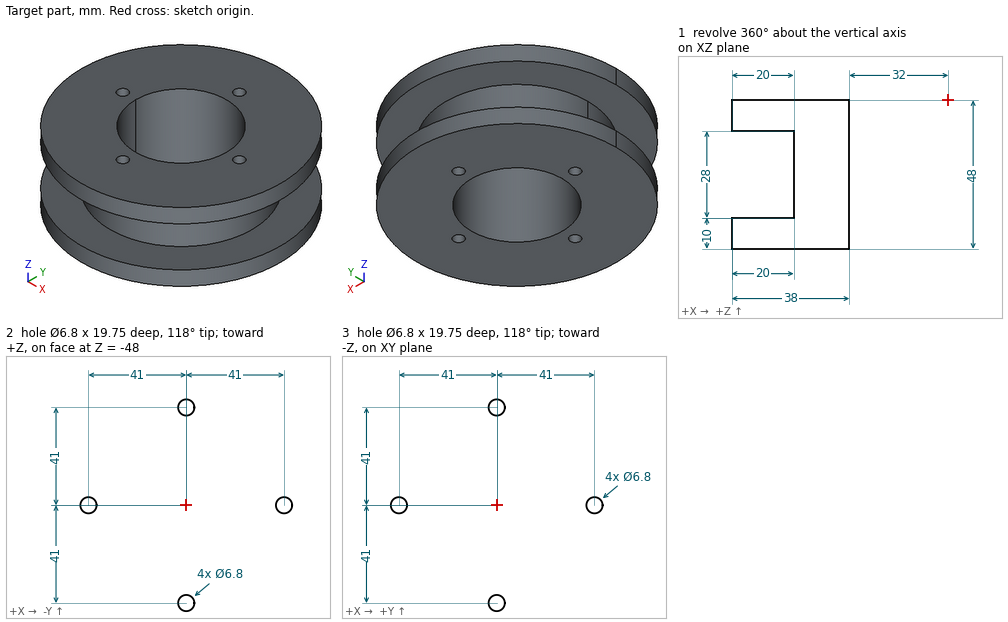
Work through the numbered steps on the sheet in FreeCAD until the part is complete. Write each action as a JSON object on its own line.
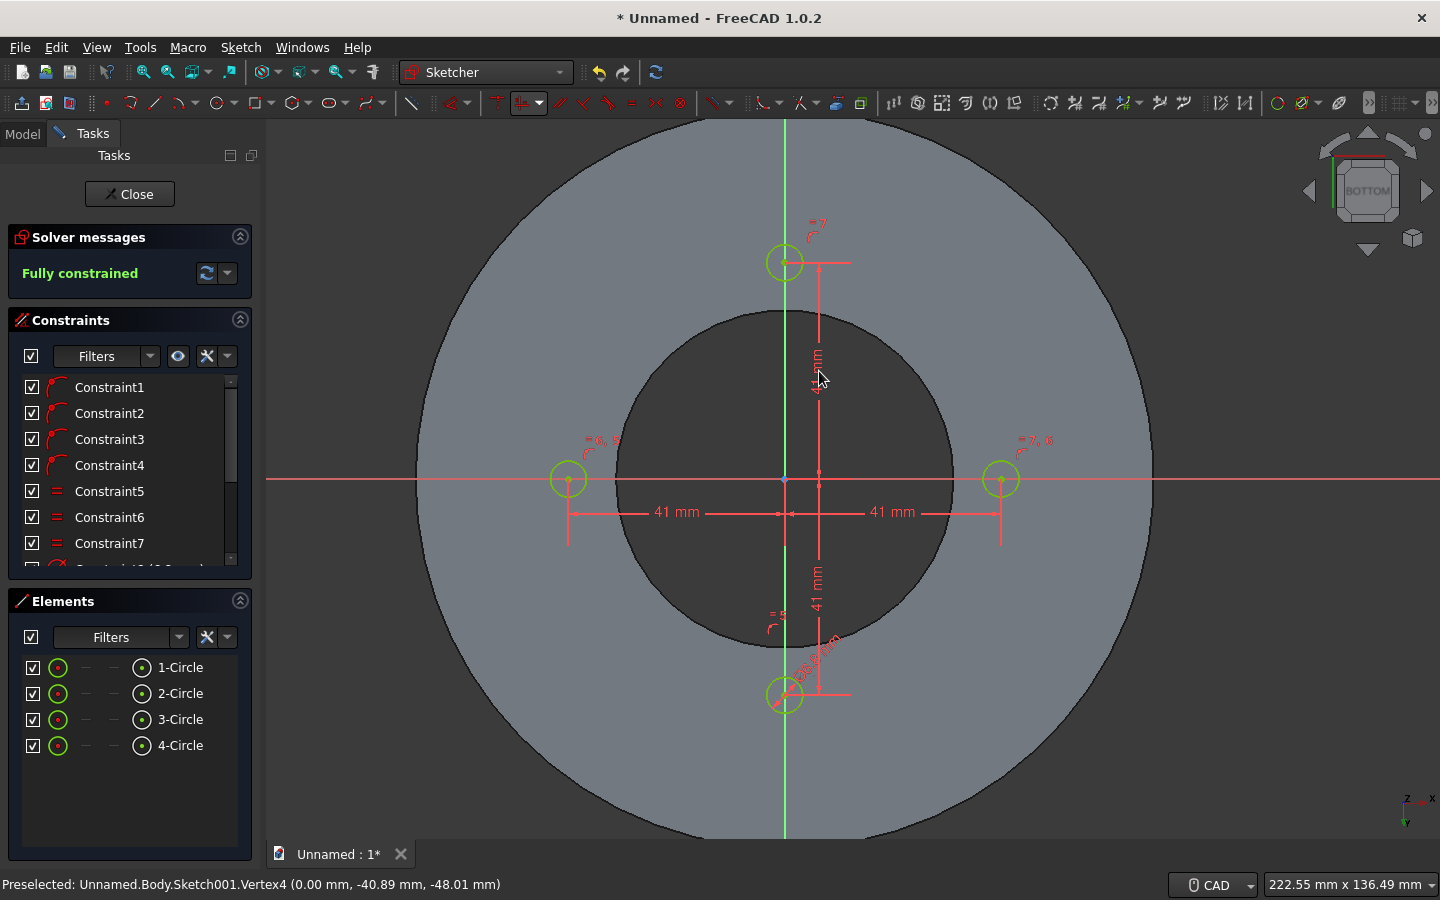
{"action": "left_click", "coordinate": [130, 194]}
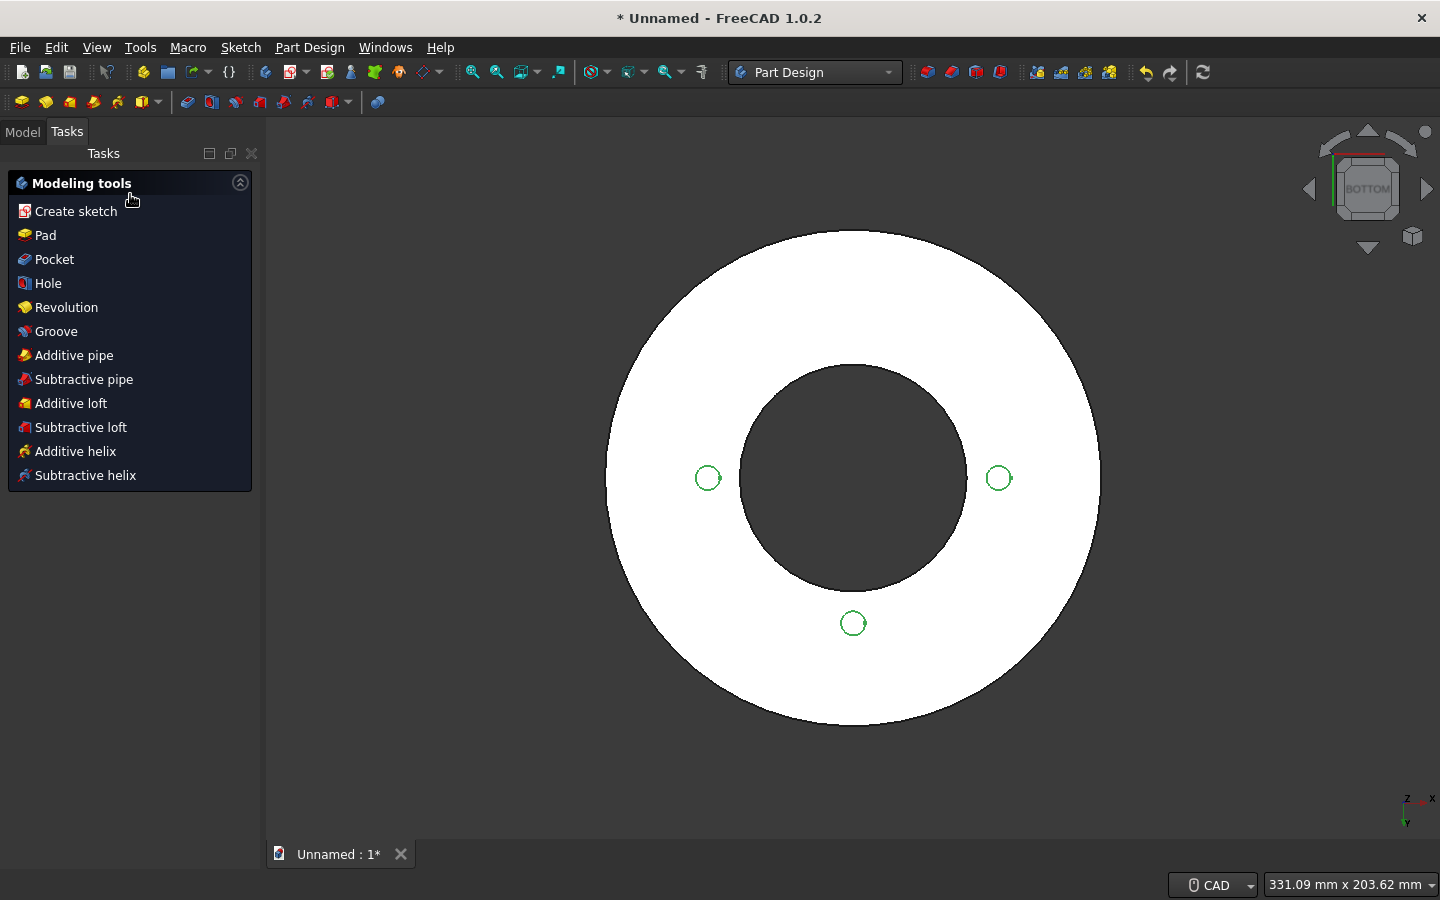
{"action": "left_click", "coordinate": [212, 102]}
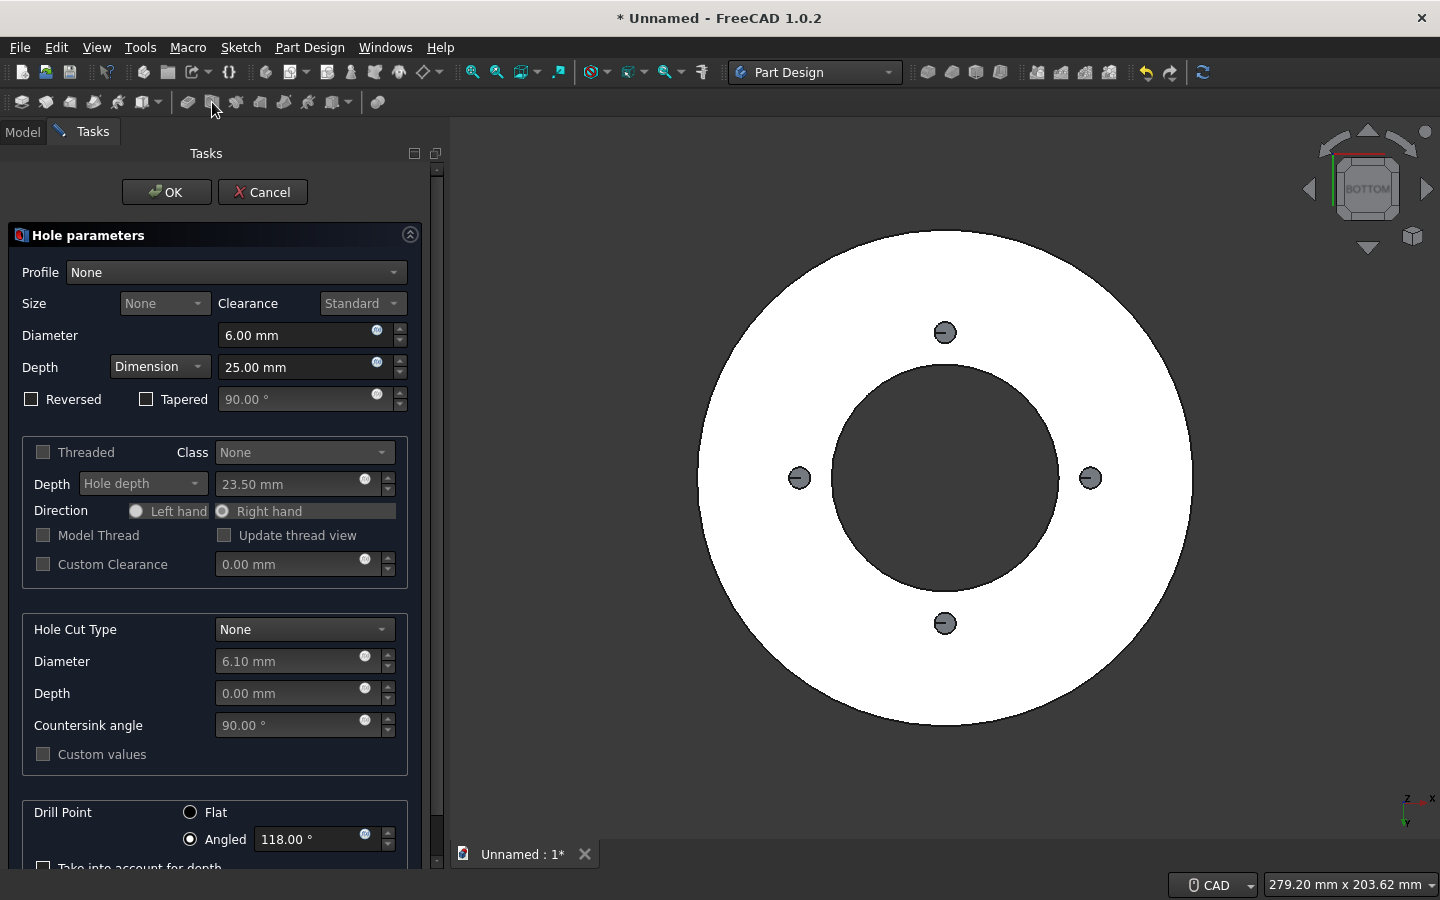
{"action": "triple_click", "coordinate": [305, 335]}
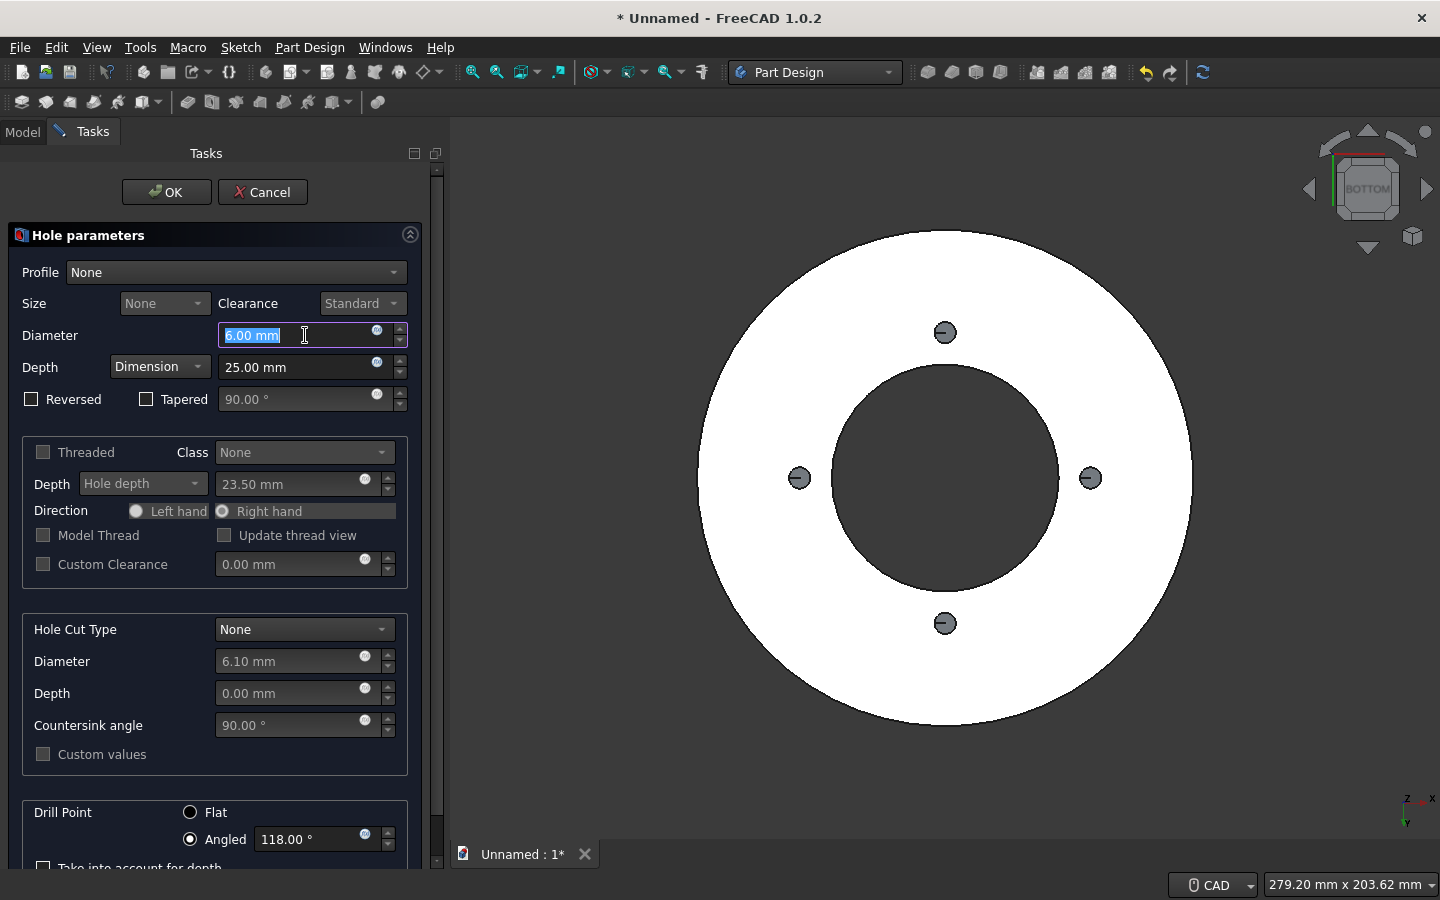
{"action": "type", "text": "6.8"}
{"action": "key", "text": "Tab"}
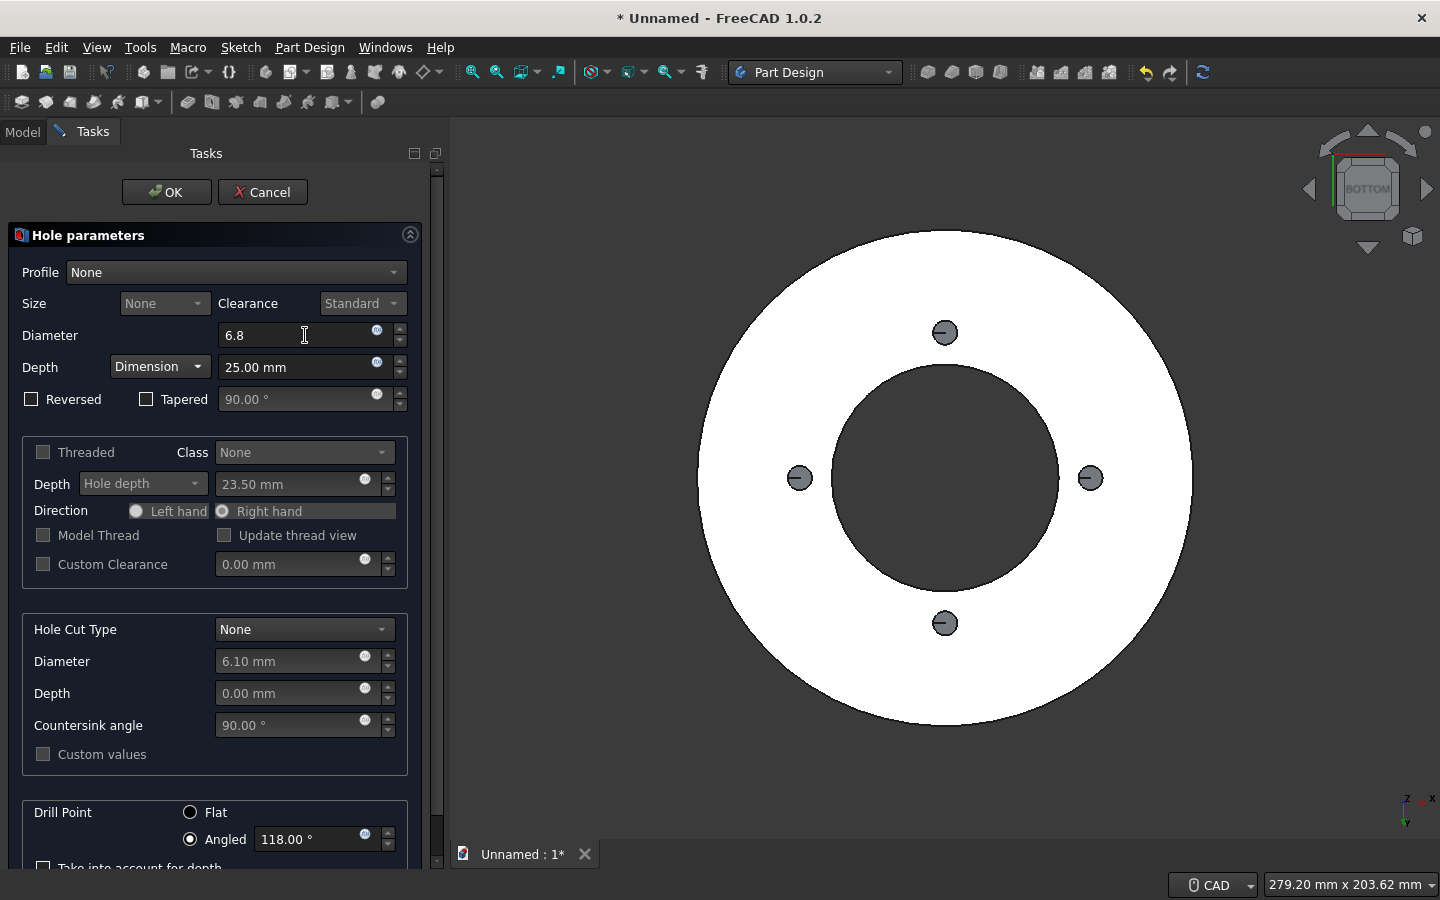
{"action": "triple_click", "coordinate": [305, 367]}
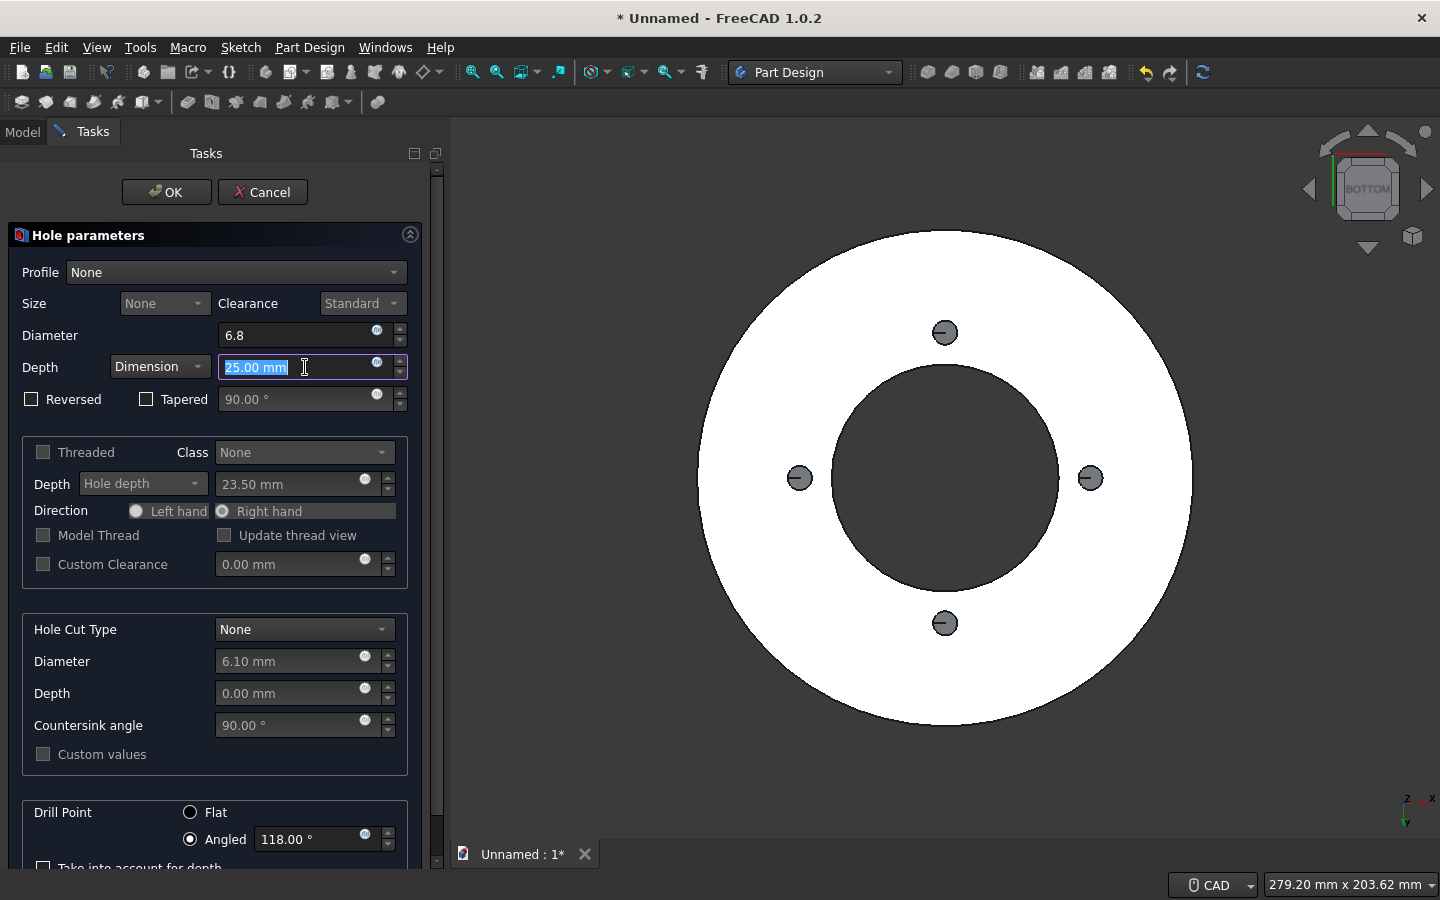
{"action": "type", "text": "19.75"}
{"action": "key", "text": "Tab"}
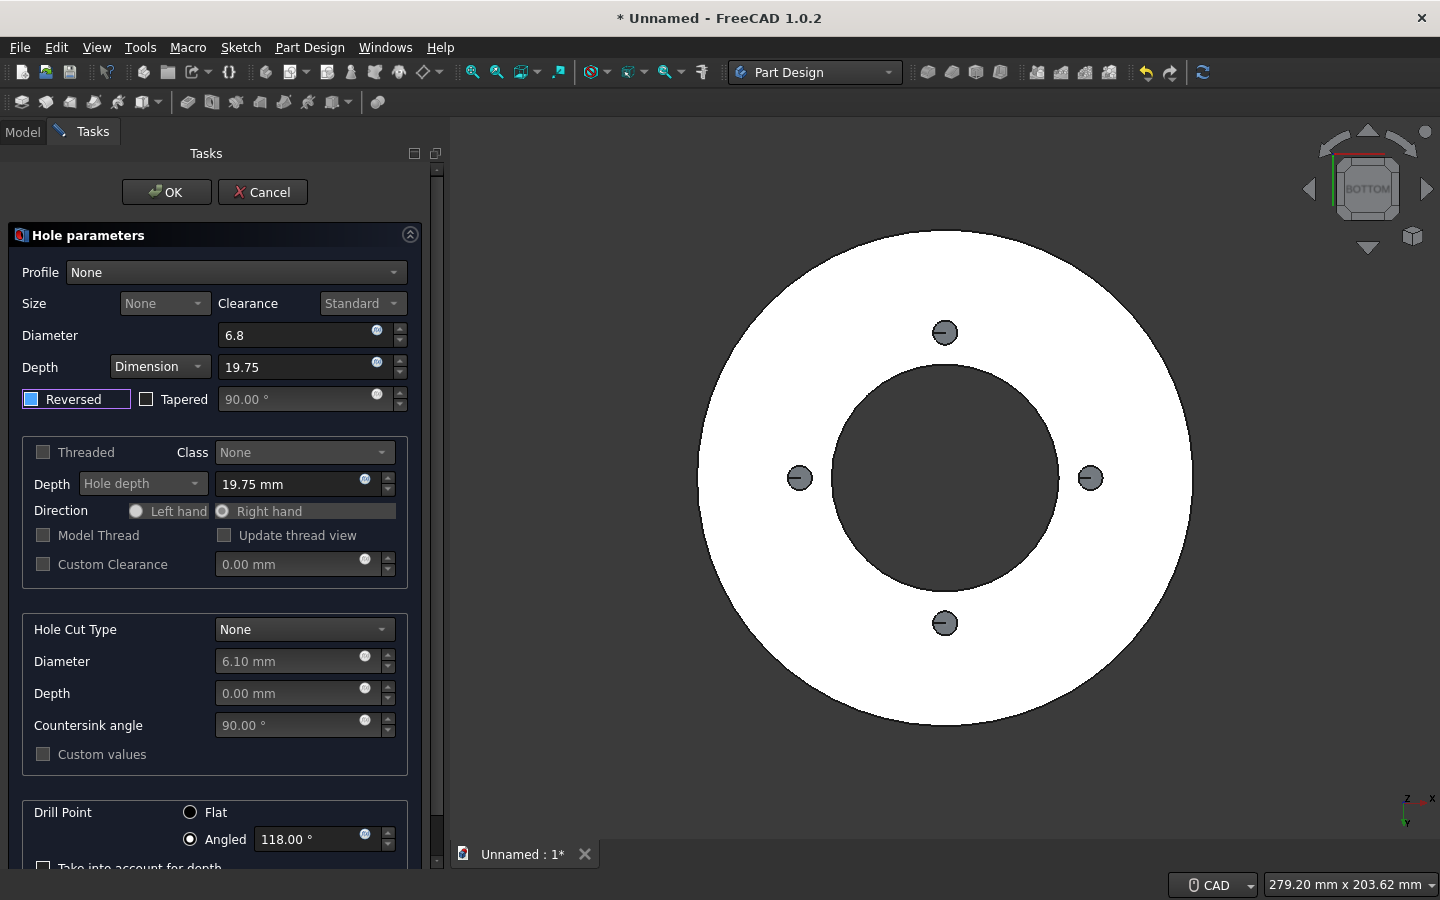
{"action": "left_click", "coordinate": [167, 192]}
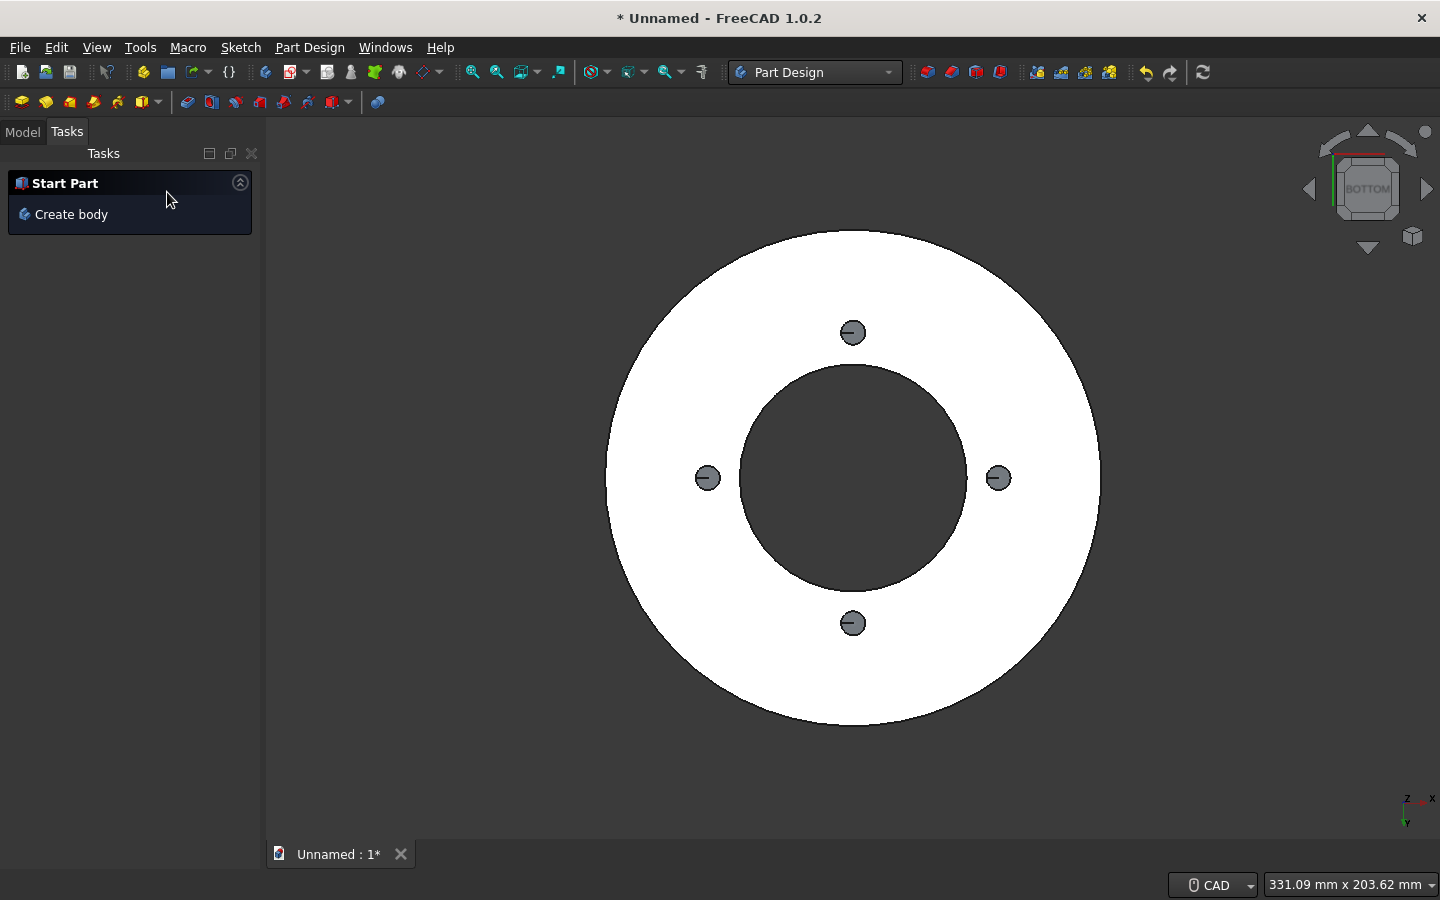
{"action": "left_click", "coordinate": [290, 72]}